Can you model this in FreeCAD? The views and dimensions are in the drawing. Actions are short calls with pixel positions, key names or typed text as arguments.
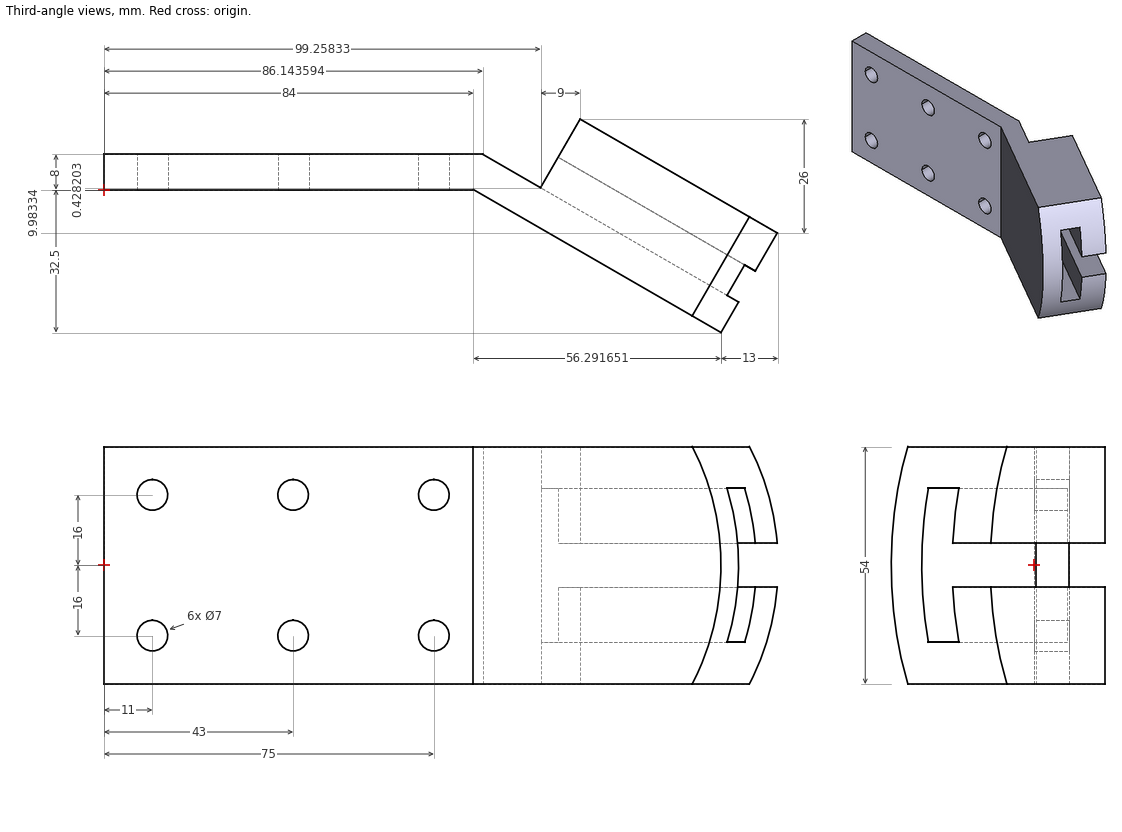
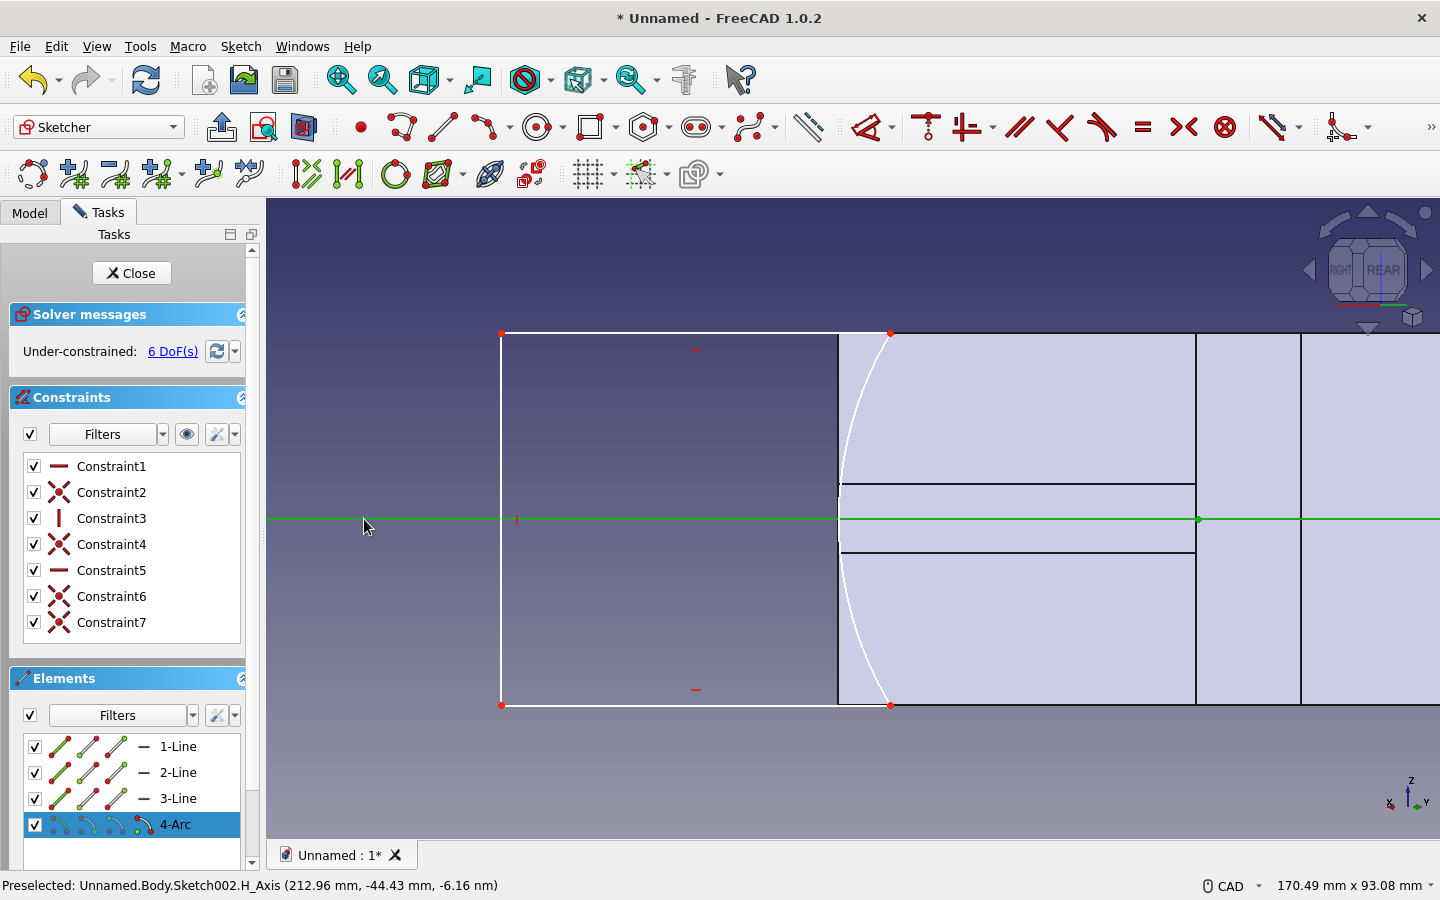
key(c)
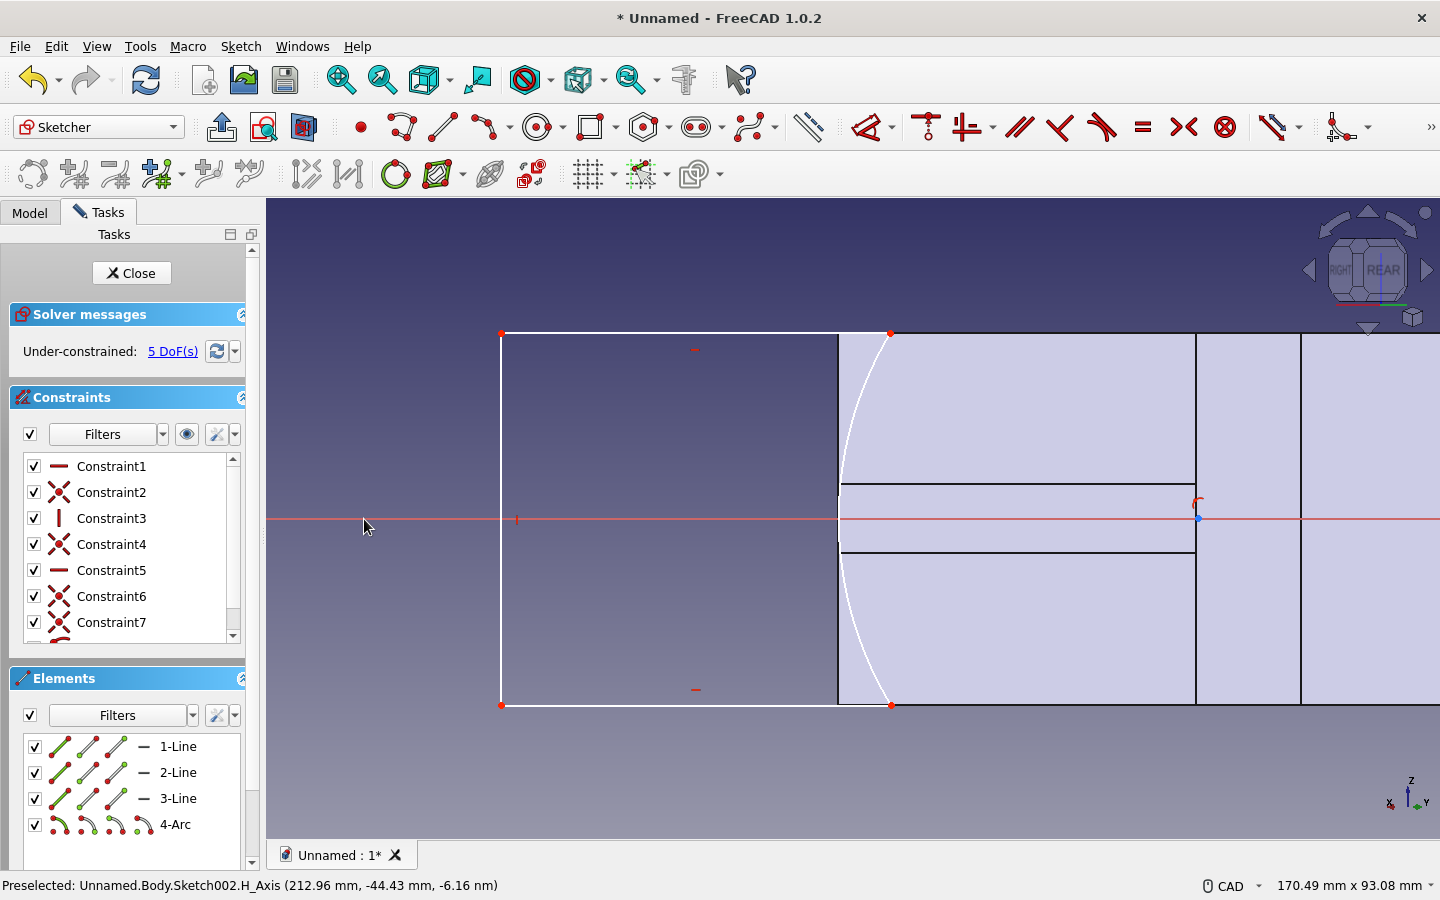
click(866, 128)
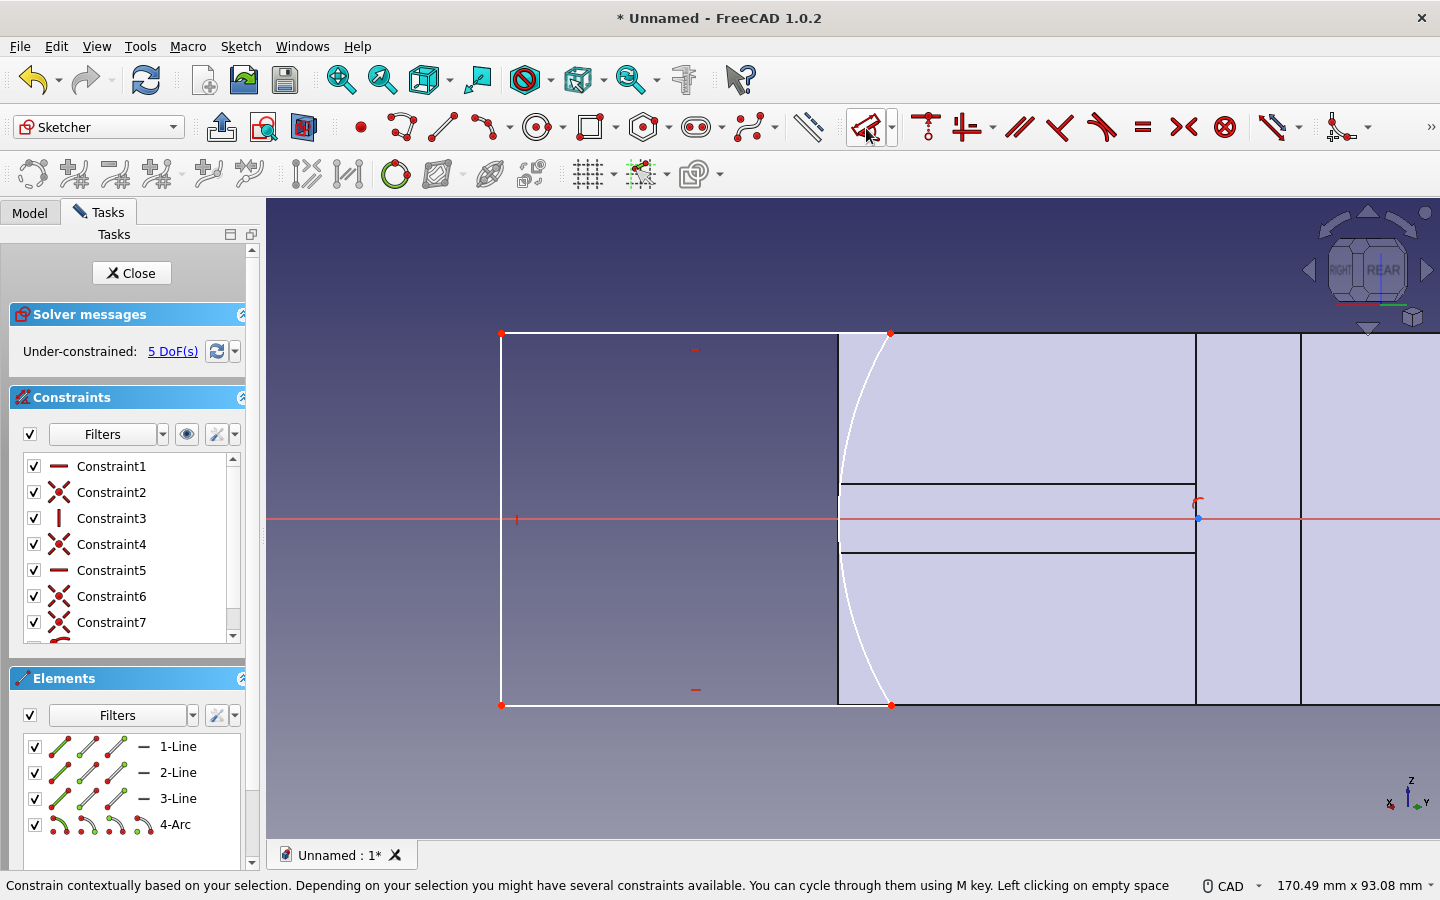
click(847, 442)
click(816, 435)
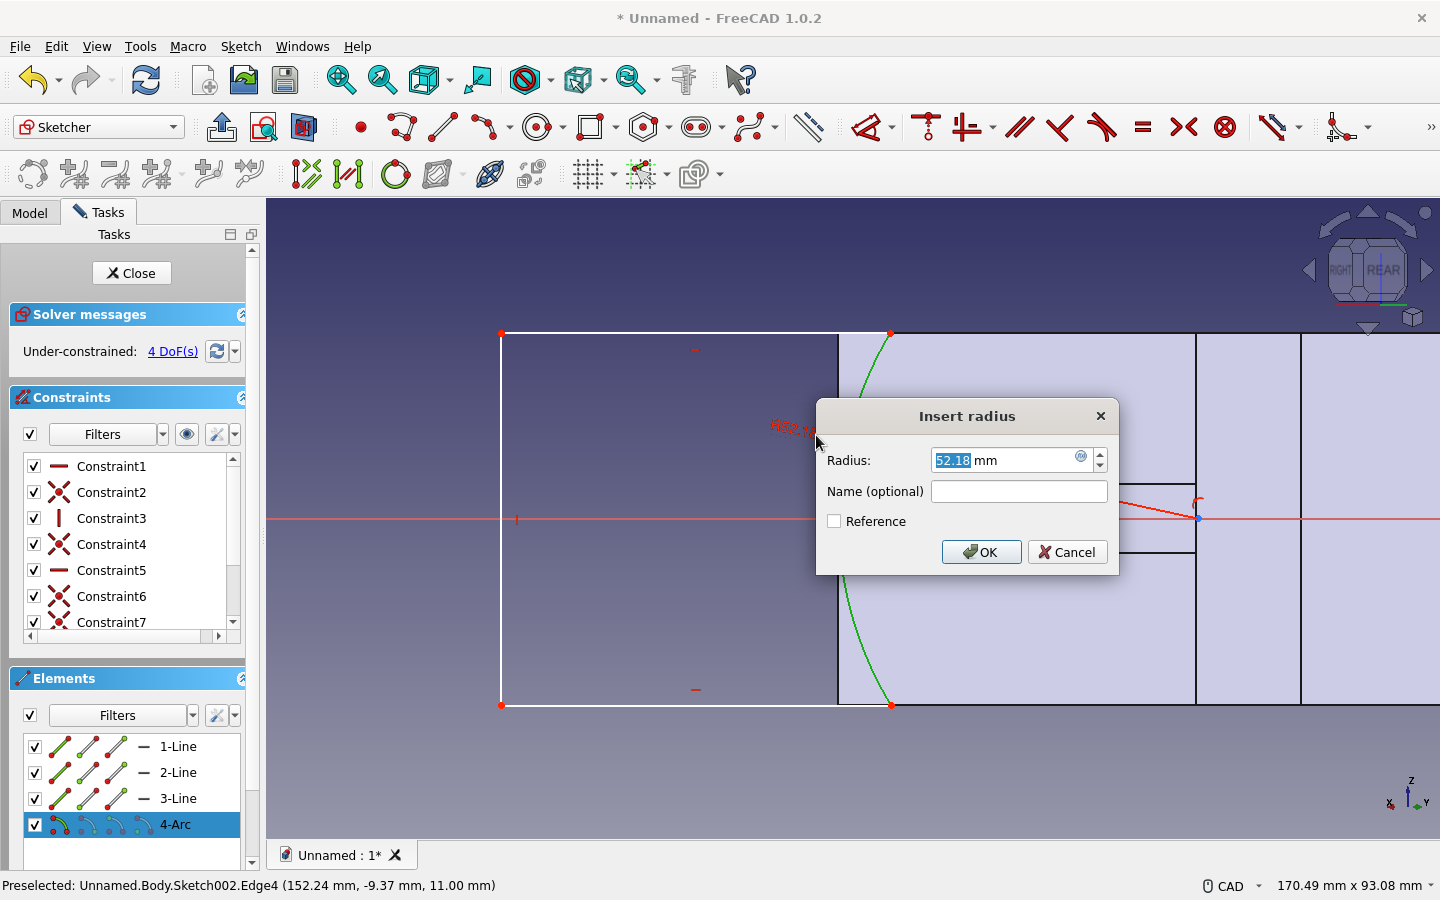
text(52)
key(Return)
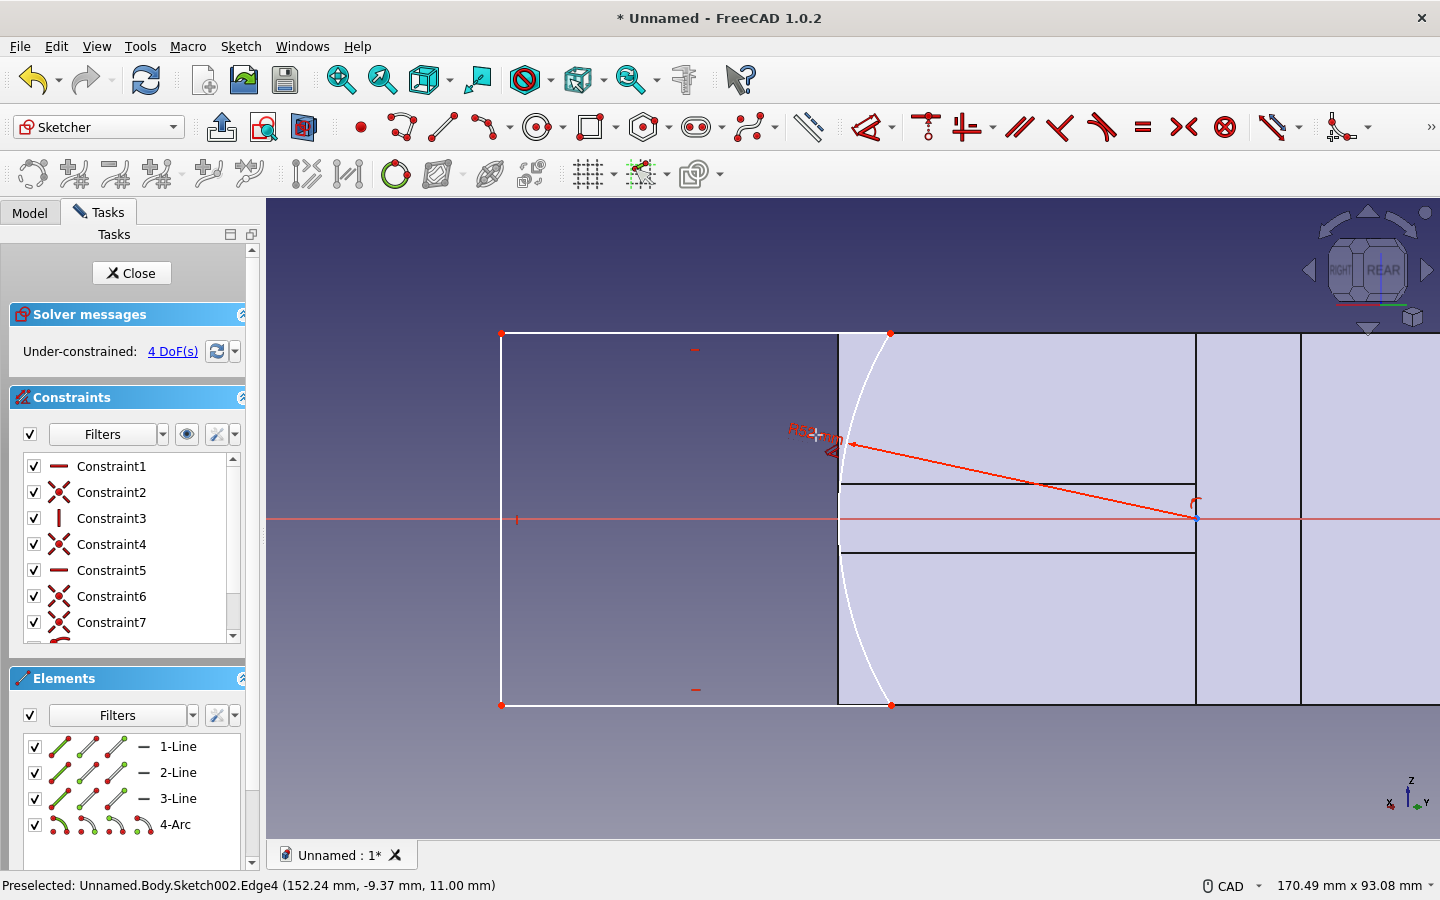
click(501, 445)
click(467, 434)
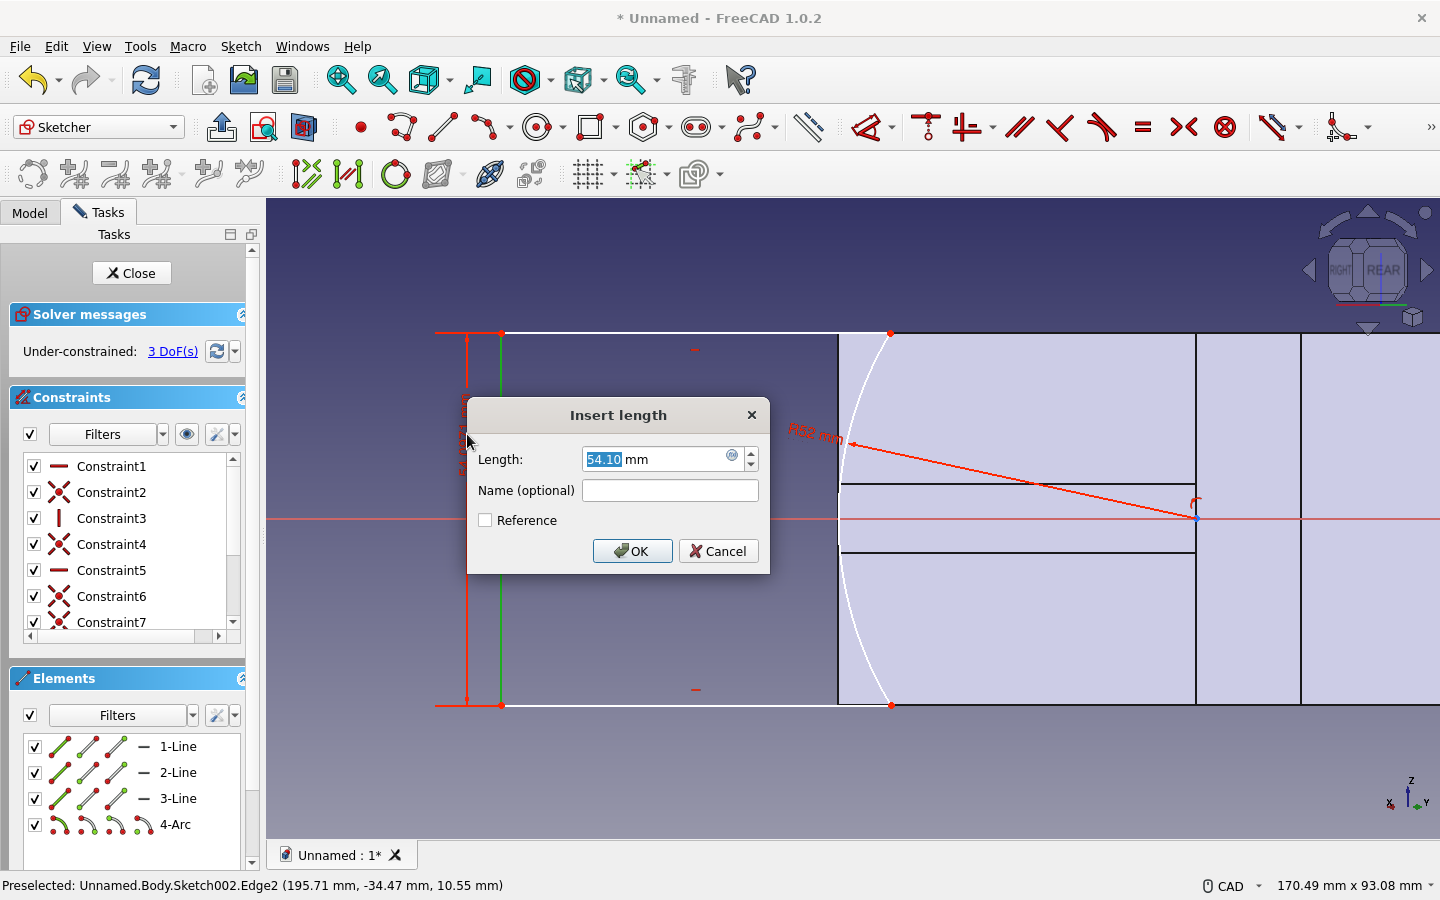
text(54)
key(Return)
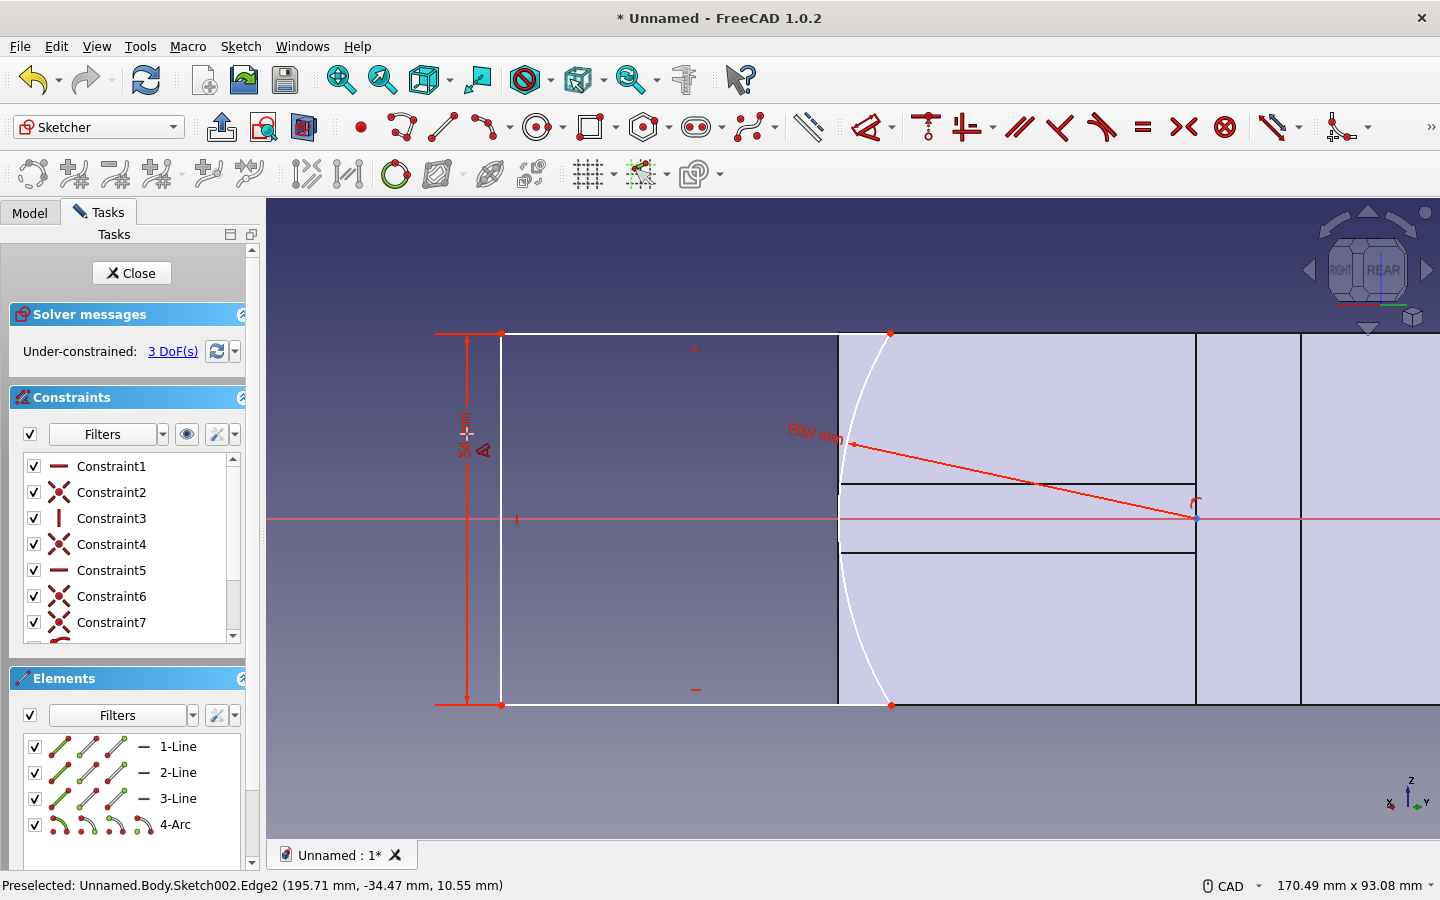
click(890, 334)
click(856, 469)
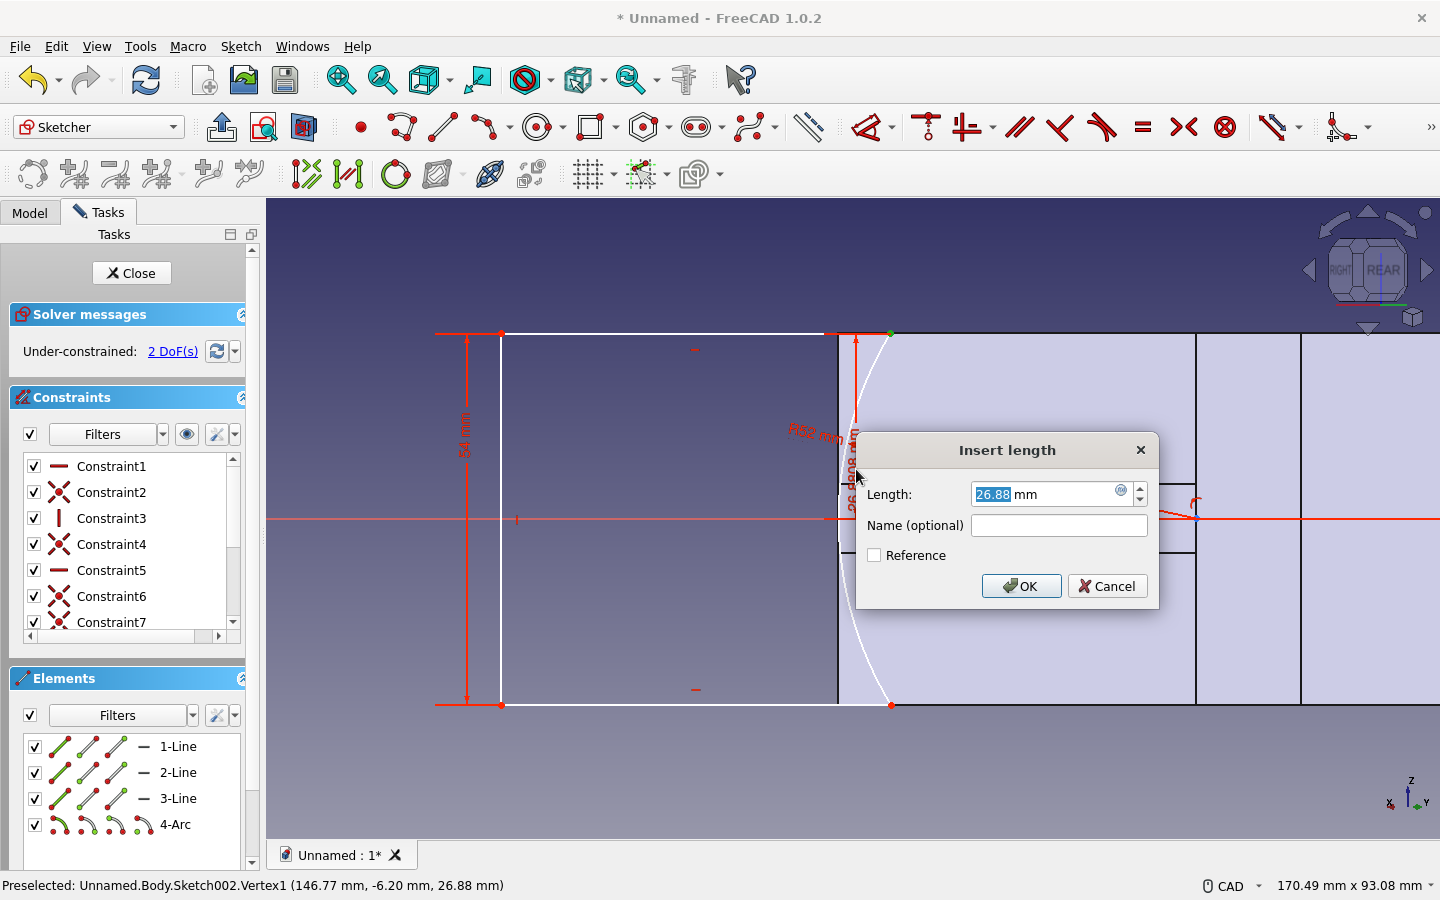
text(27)
key(Return)